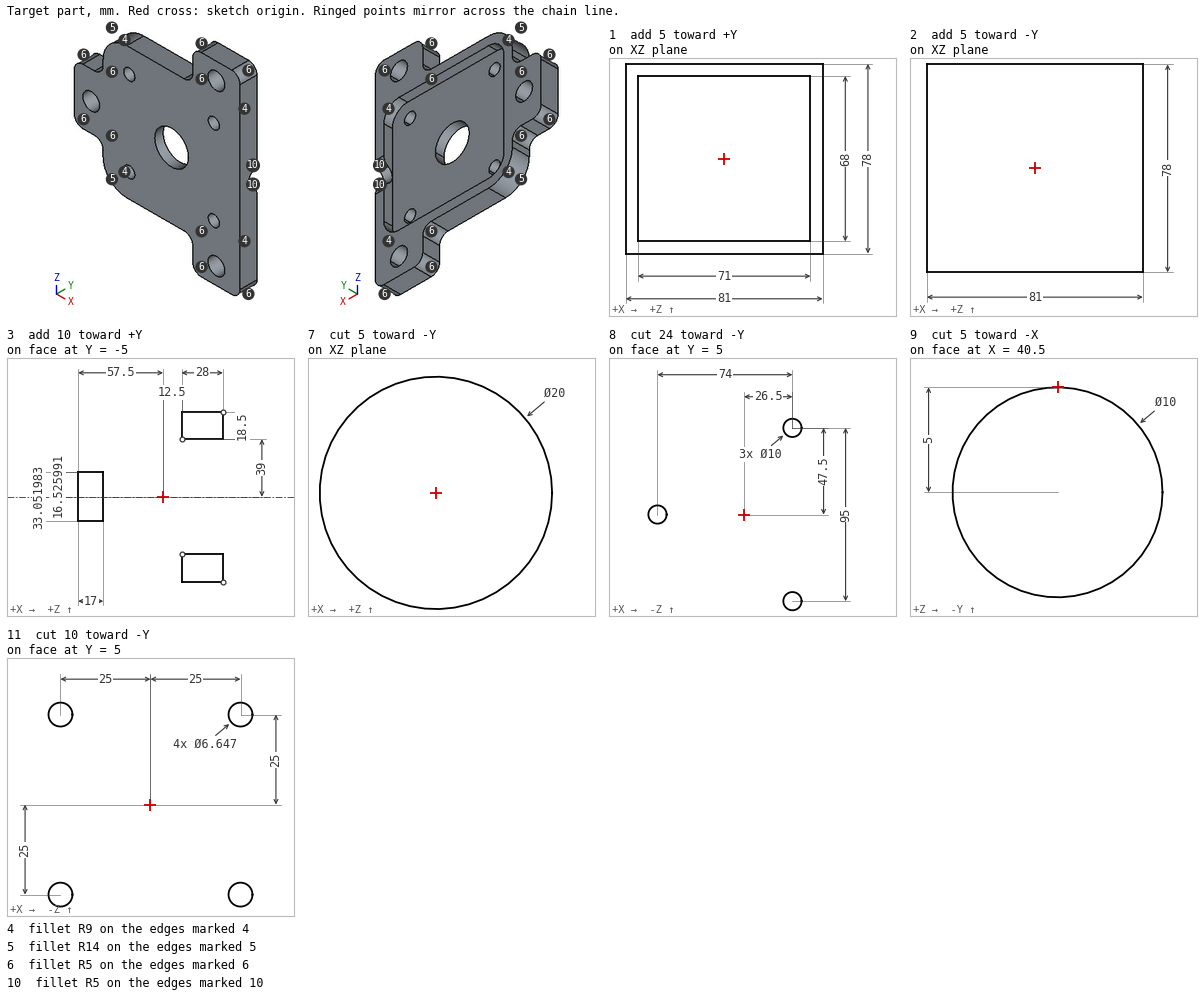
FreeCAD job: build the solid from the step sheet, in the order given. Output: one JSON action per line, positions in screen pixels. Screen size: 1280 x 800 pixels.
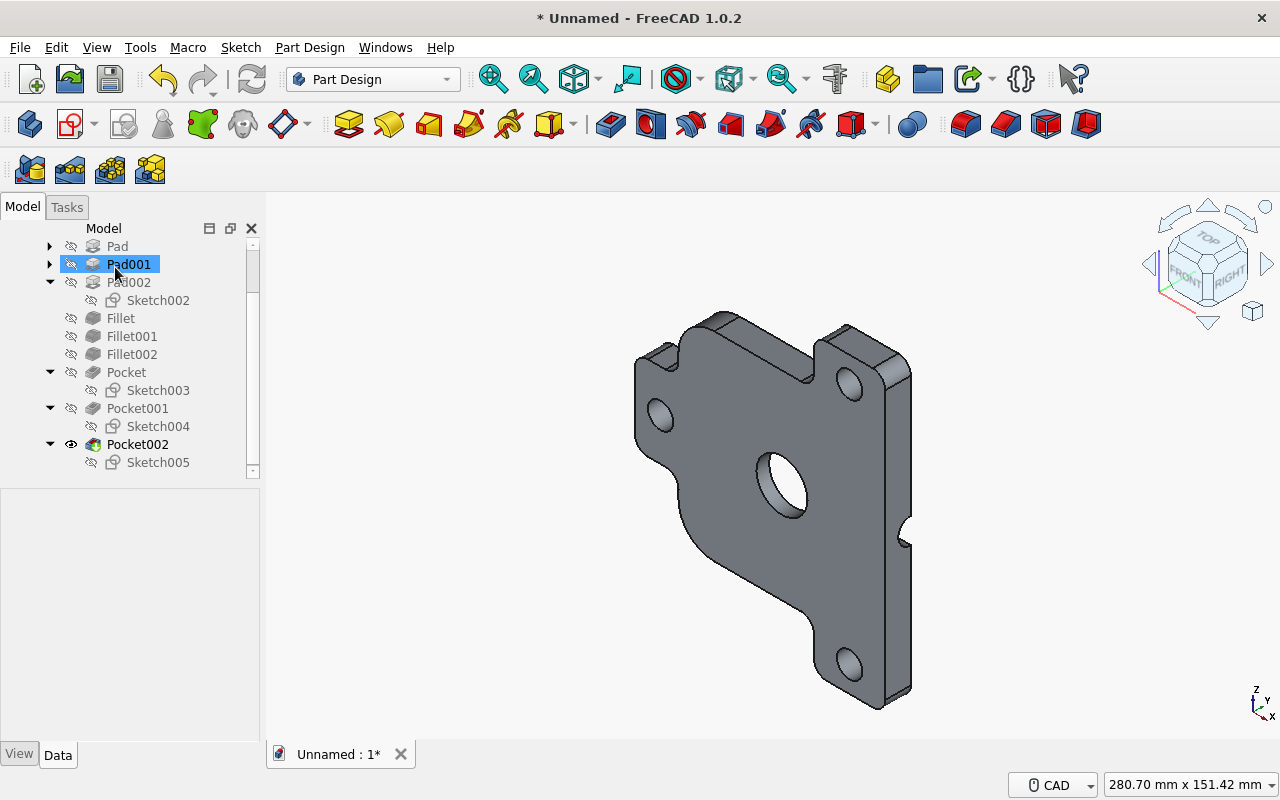
{"action": "scroll", "coordinate": [905, 511], "scroll_direction": "up", "scroll_amount": 4}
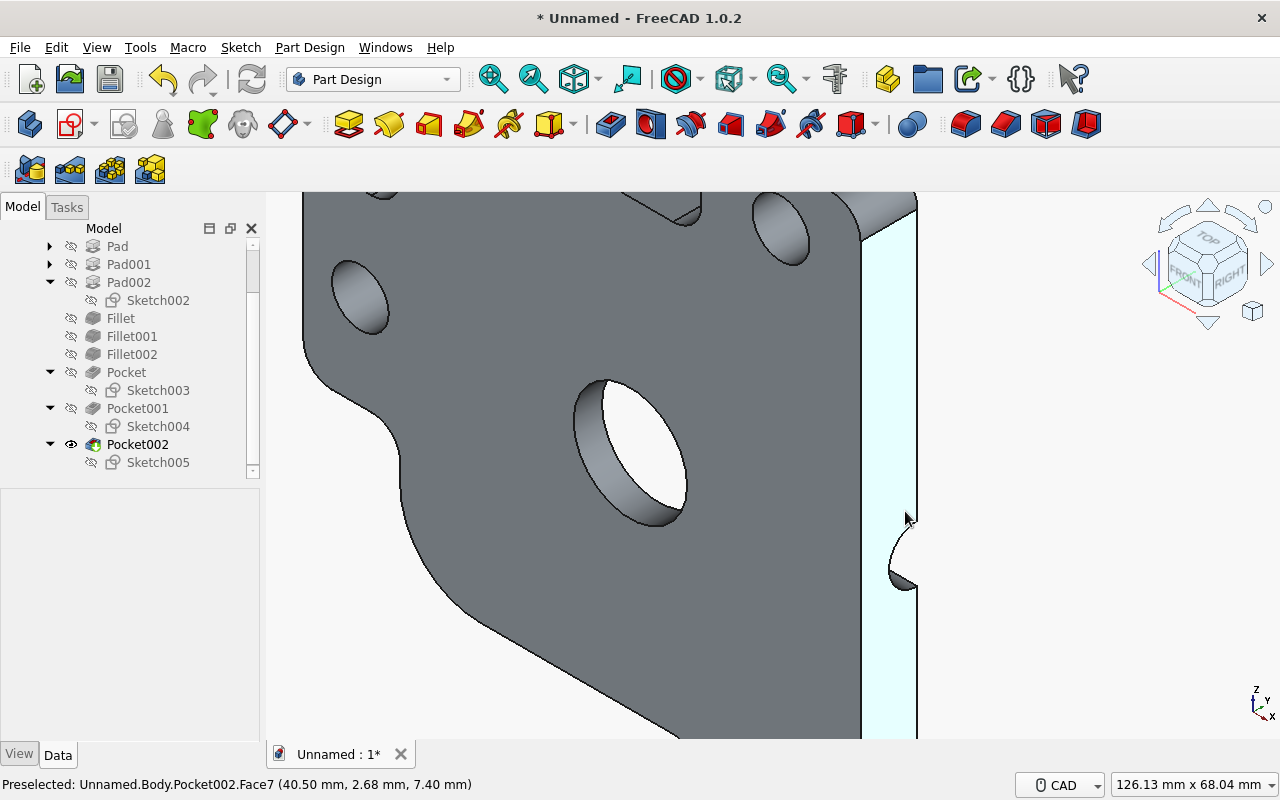
{"action": "left_click", "coordinate": [494, 80]}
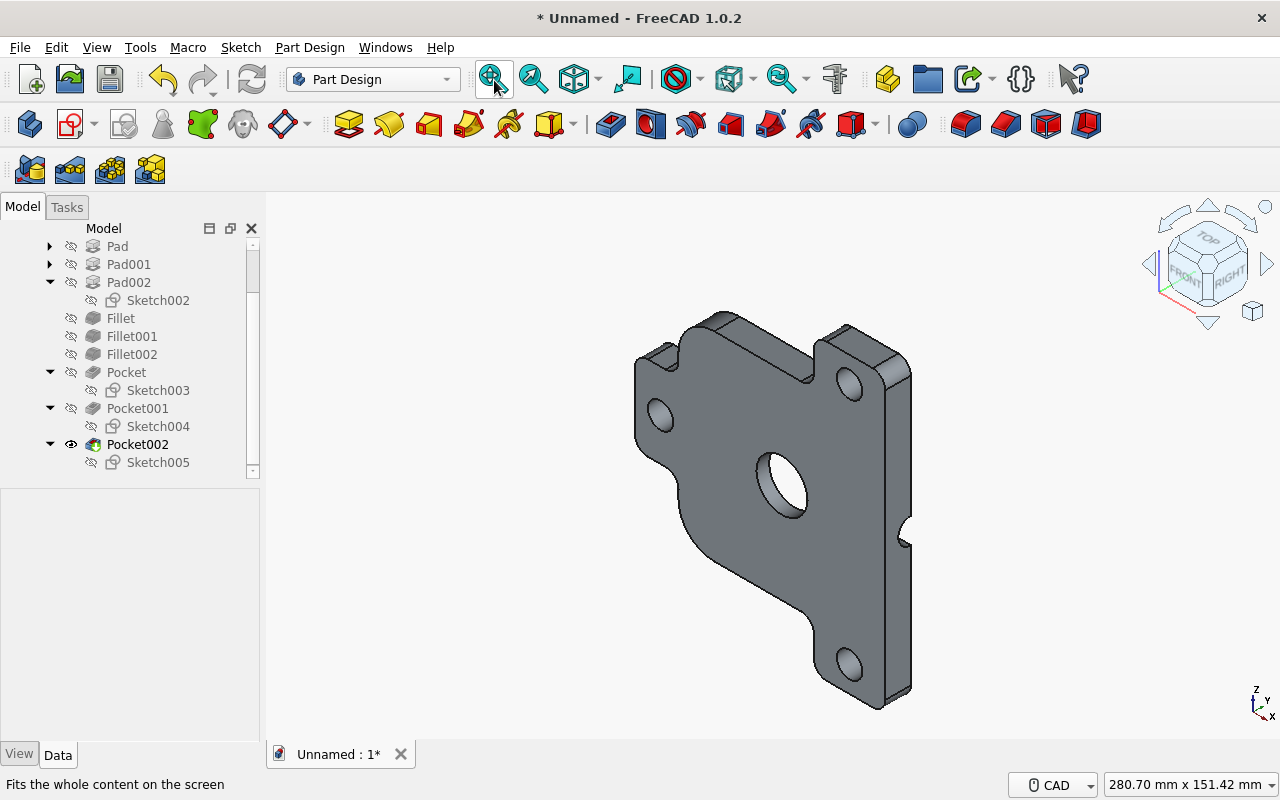
{"action": "key", "text": "2"}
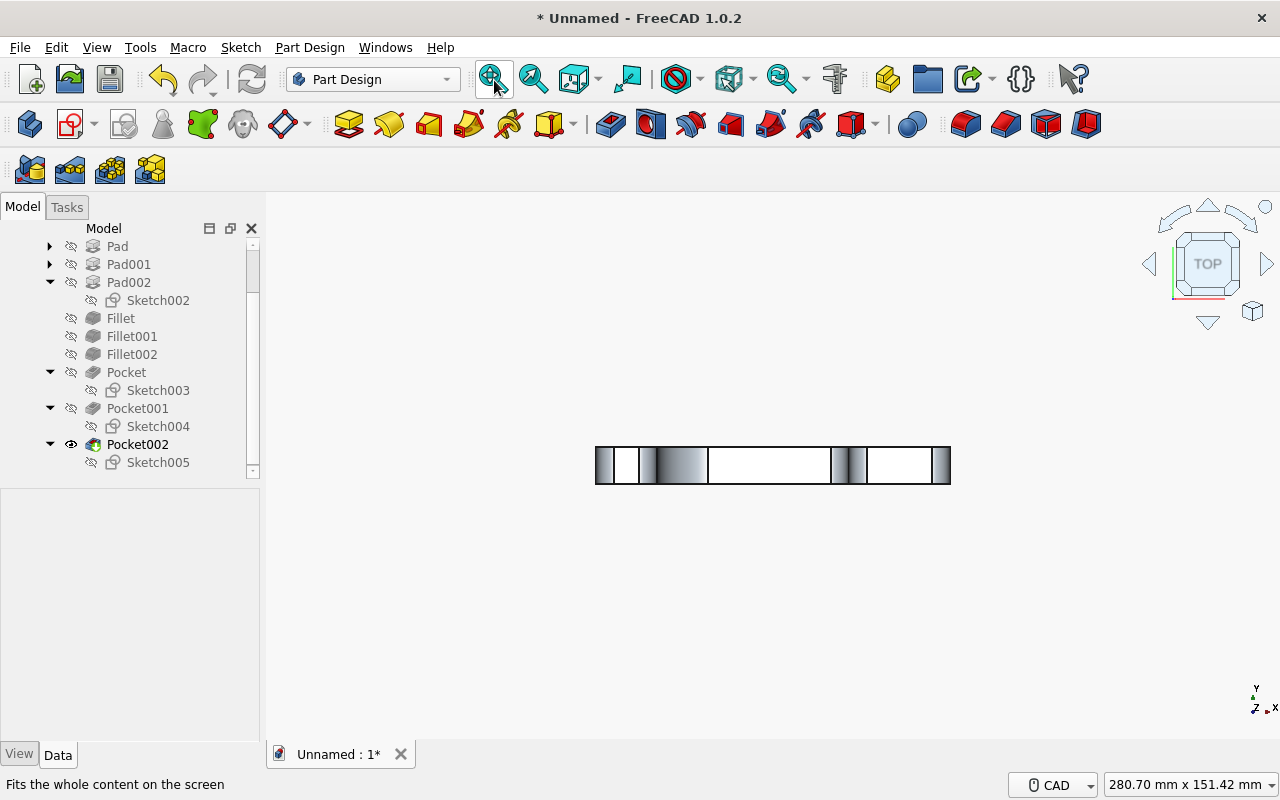
{"action": "key", "text": "v f"}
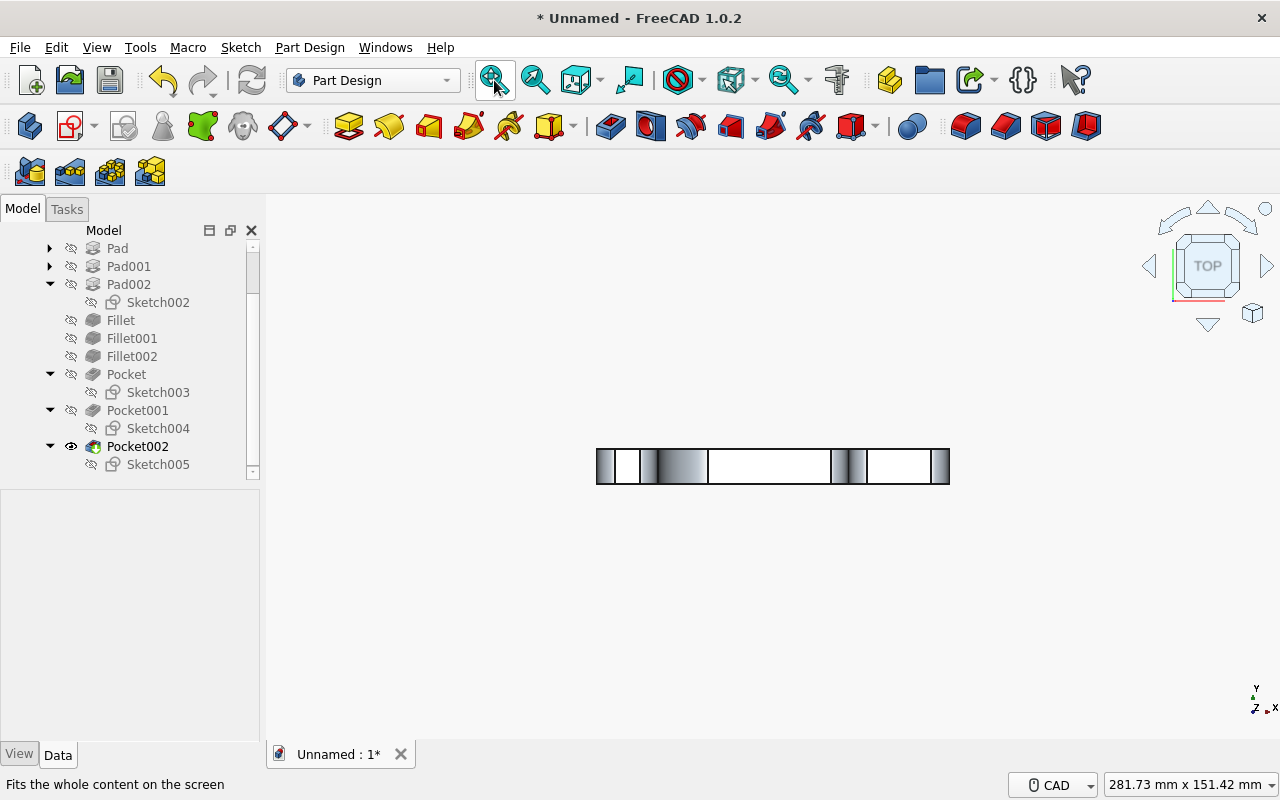
{"action": "scroll", "coordinate": [940, 448], "scroll_direction": "up", "scroll_amount": 4}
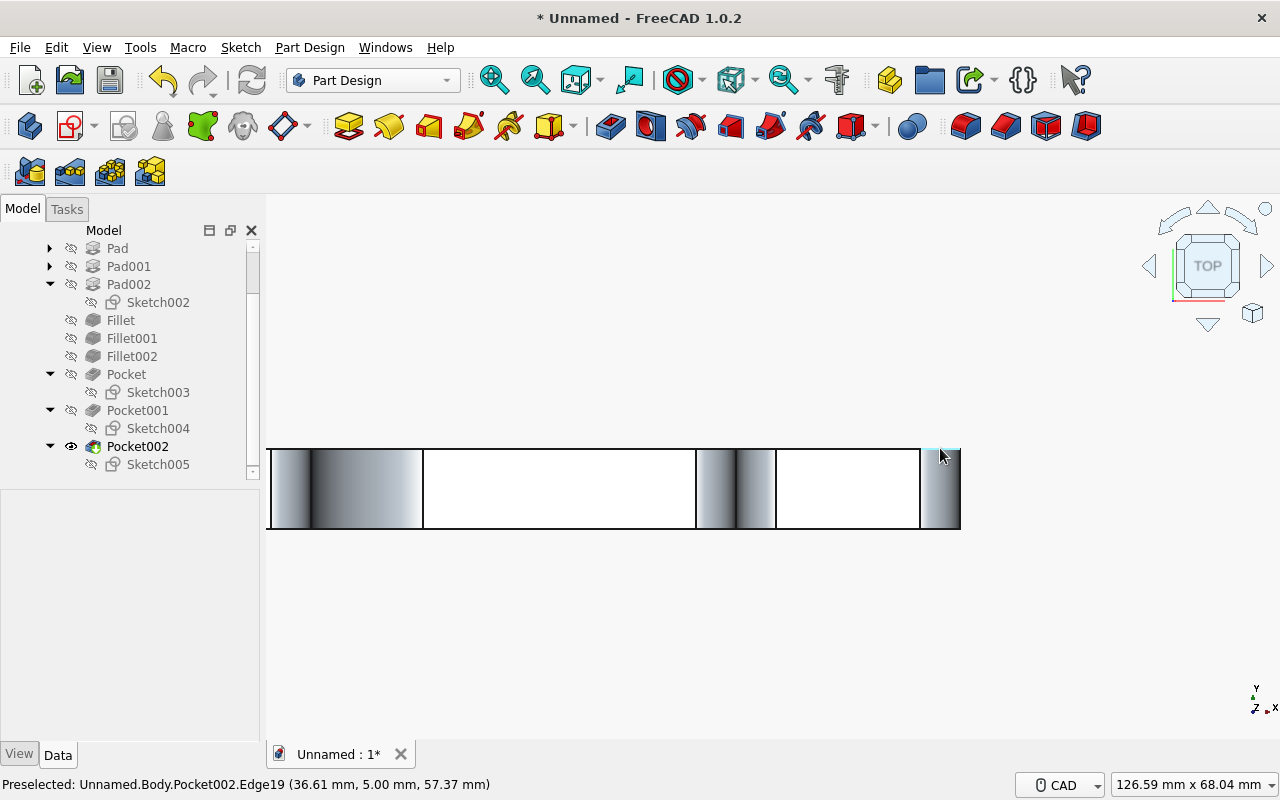
{"action": "left_click", "coordinate": [496, 80]}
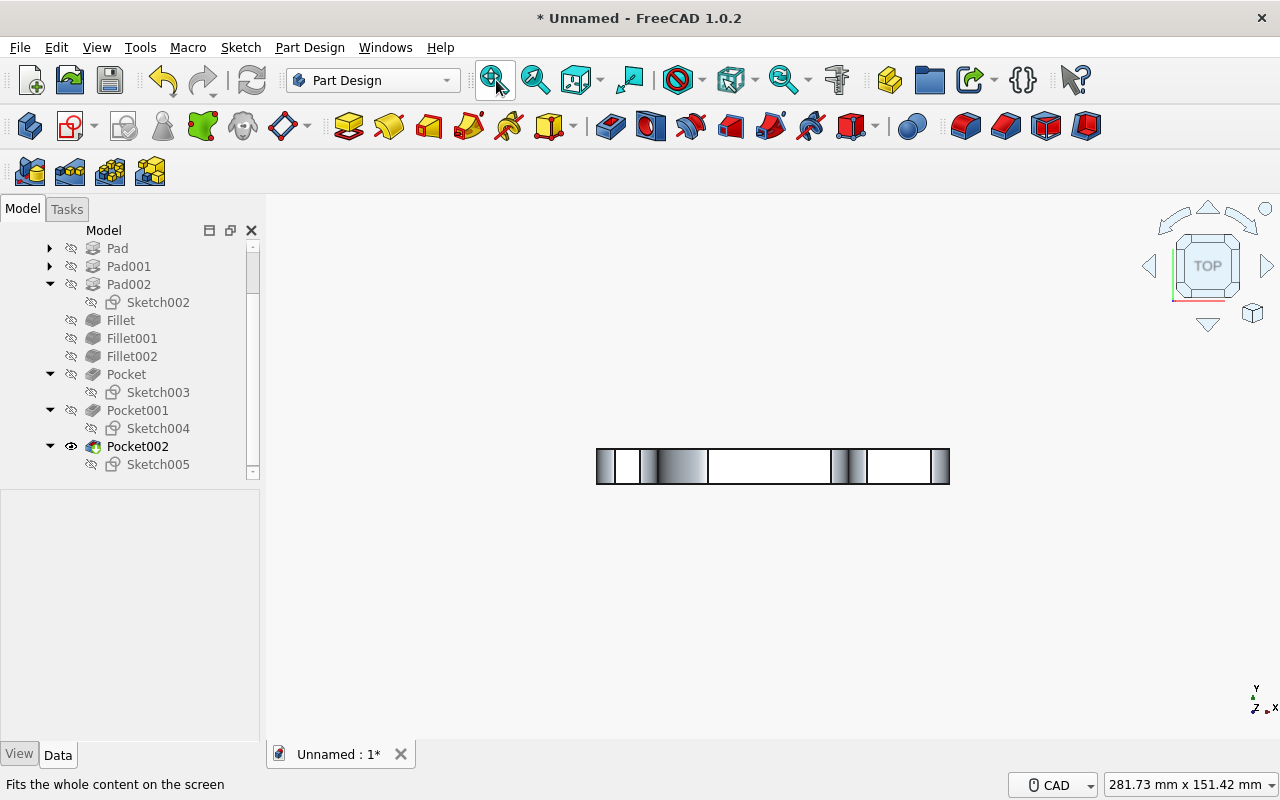
{"action": "key", "text": "0"}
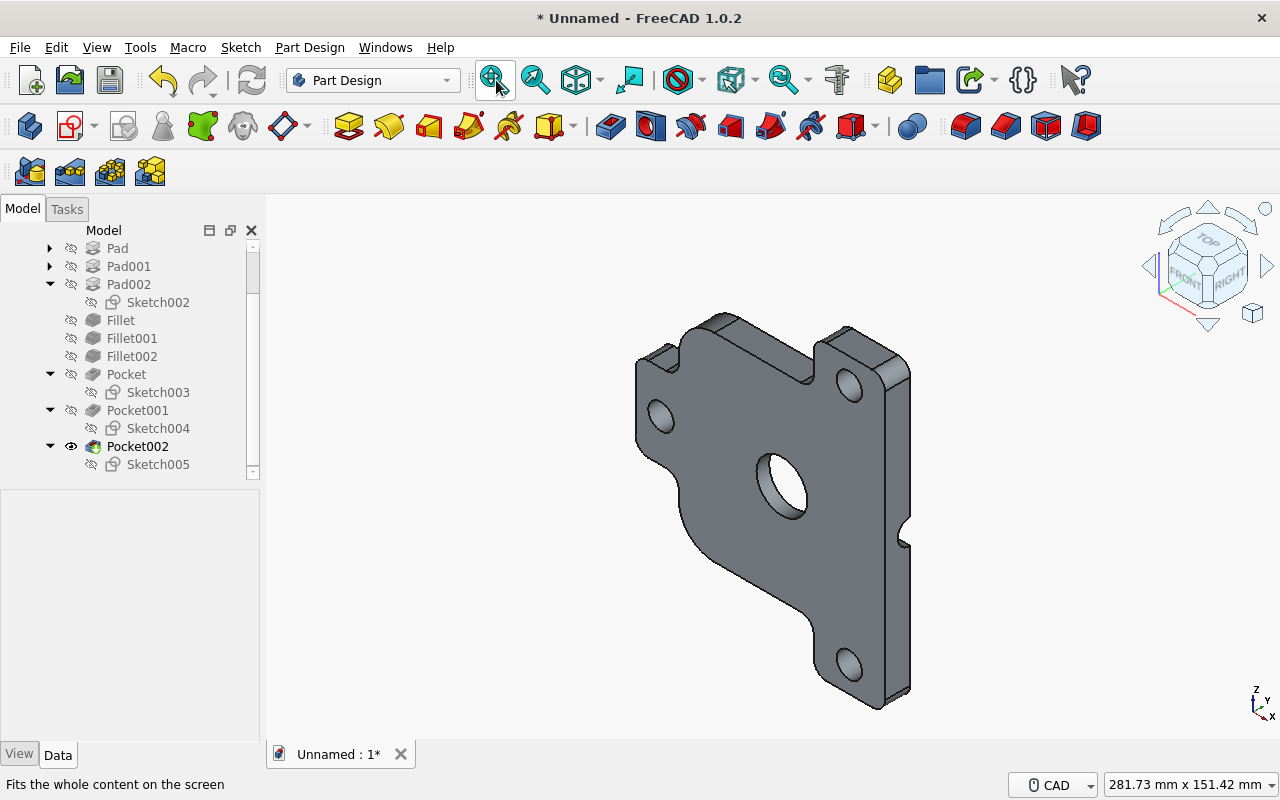
{"action": "scroll", "coordinate": [904, 512], "scroll_direction": "up", "scroll_amount": 4}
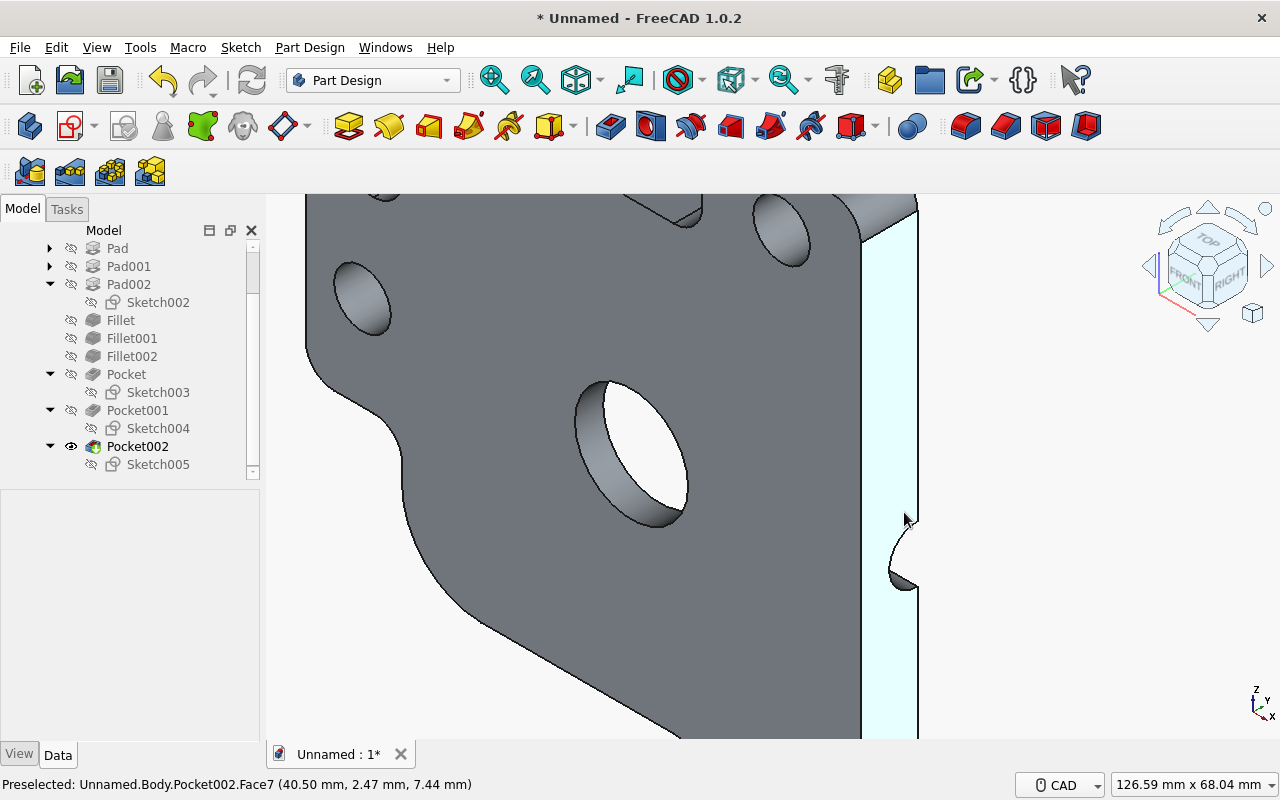
{"action": "left_click", "coordinate": [496, 80]}